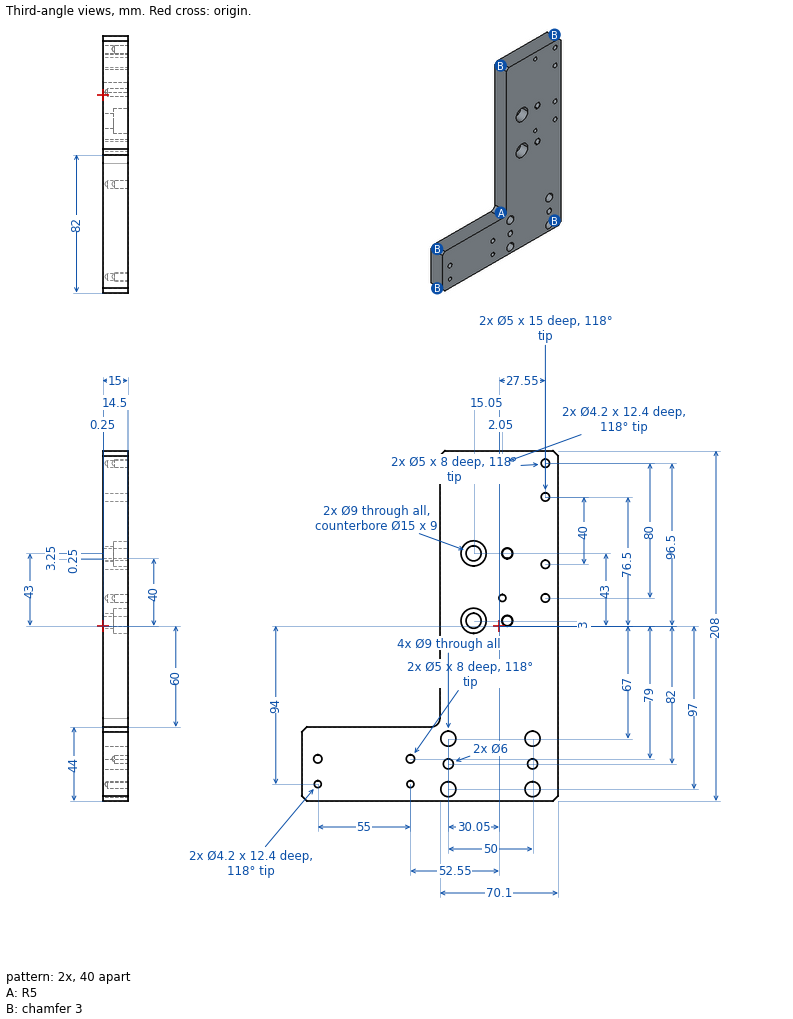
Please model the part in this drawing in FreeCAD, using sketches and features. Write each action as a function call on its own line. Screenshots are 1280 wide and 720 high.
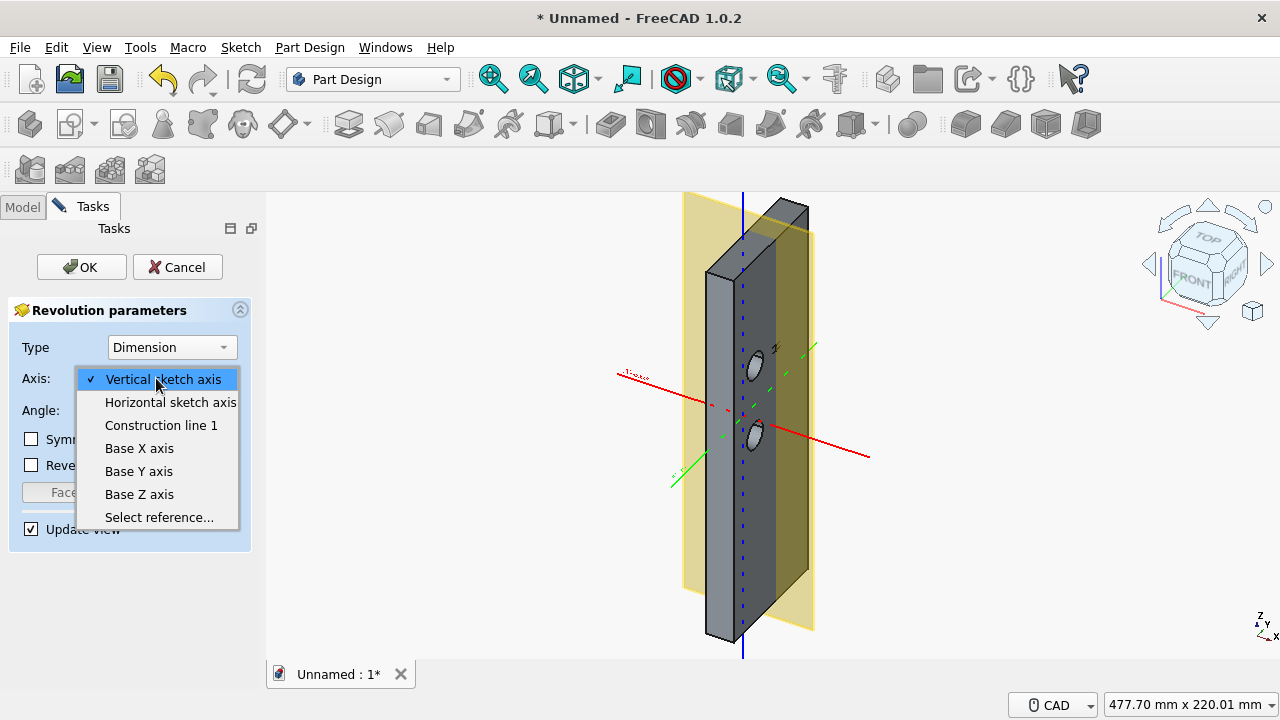
click(156, 426)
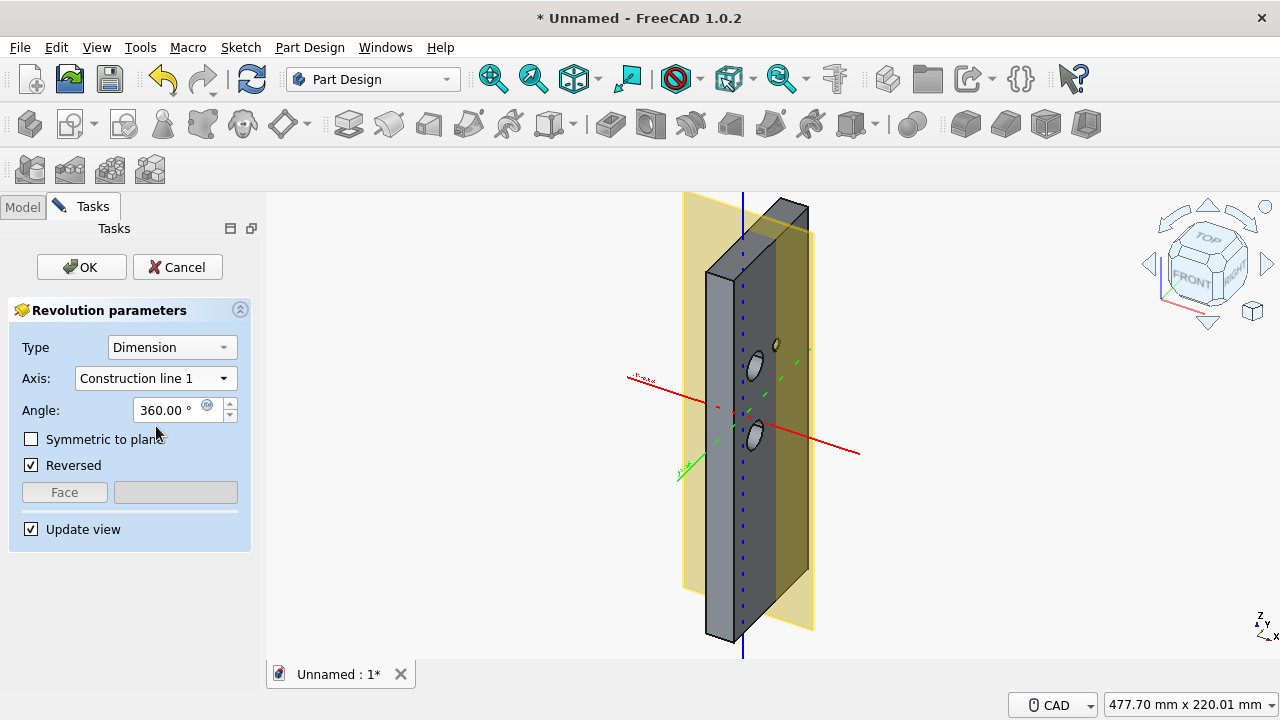
click(82, 267)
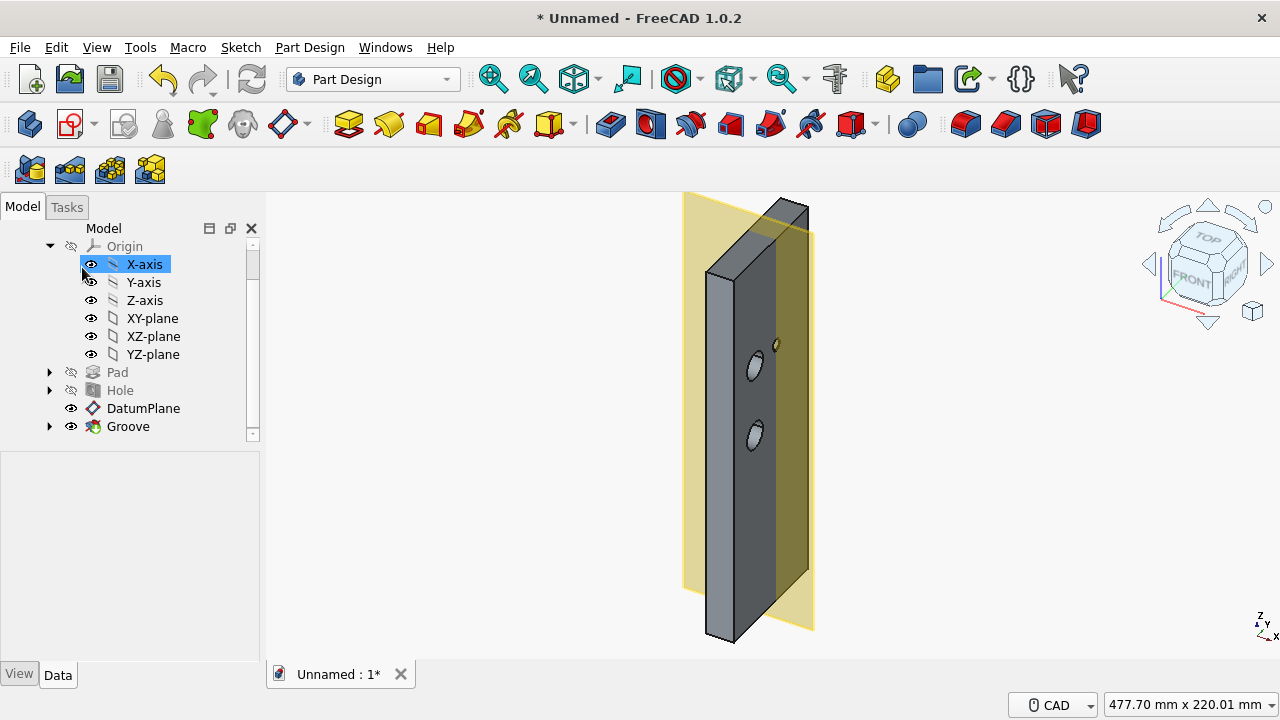
click(116, 408)
key(space)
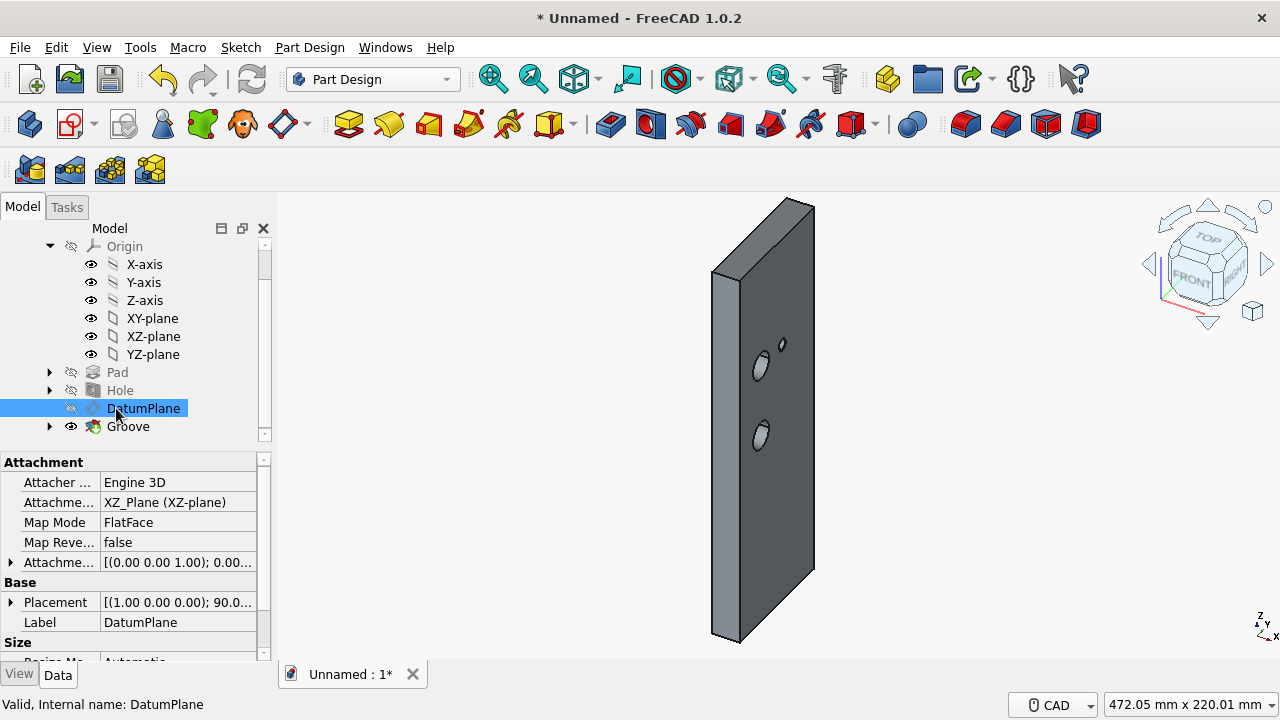
click(116, 426)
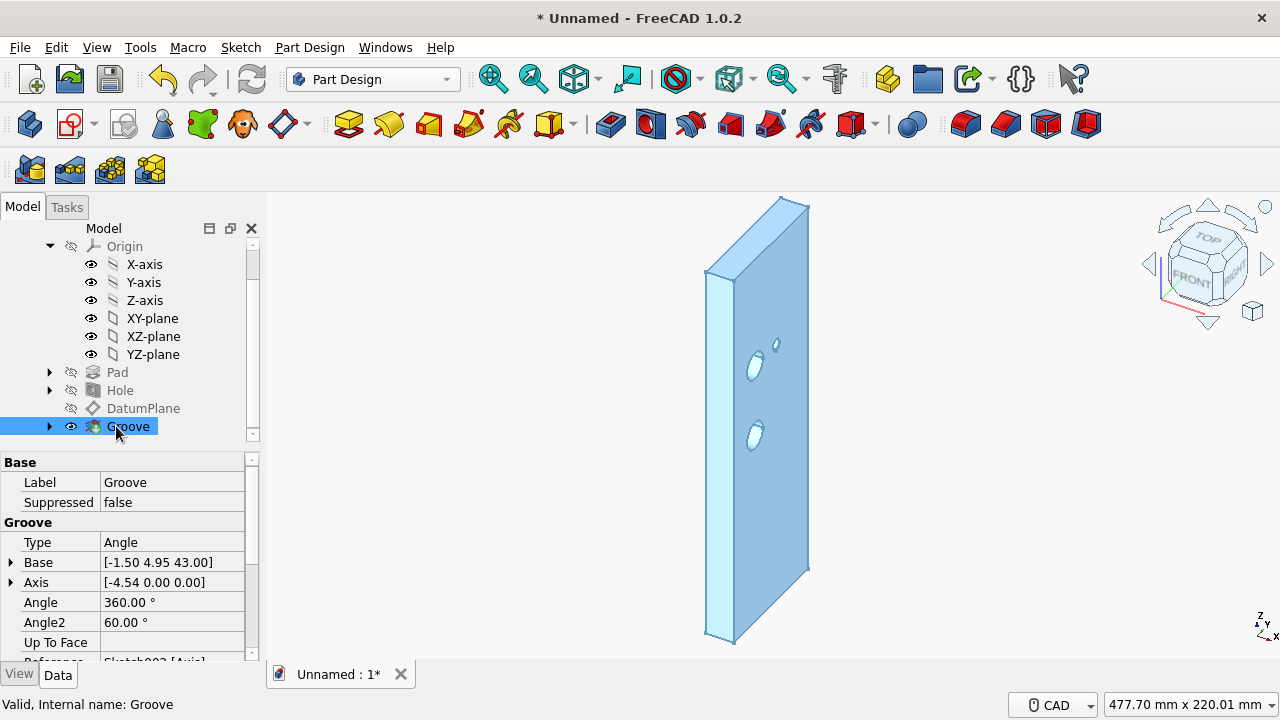
click(70, 170)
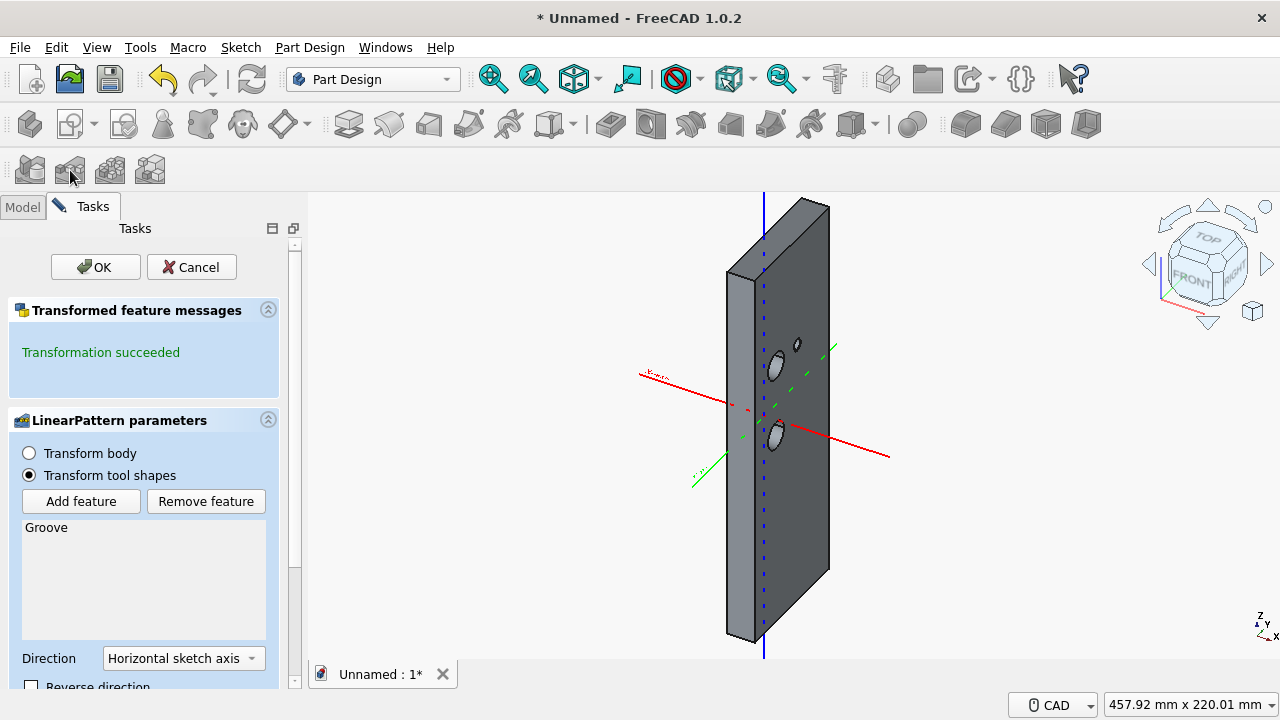
click(184, 658)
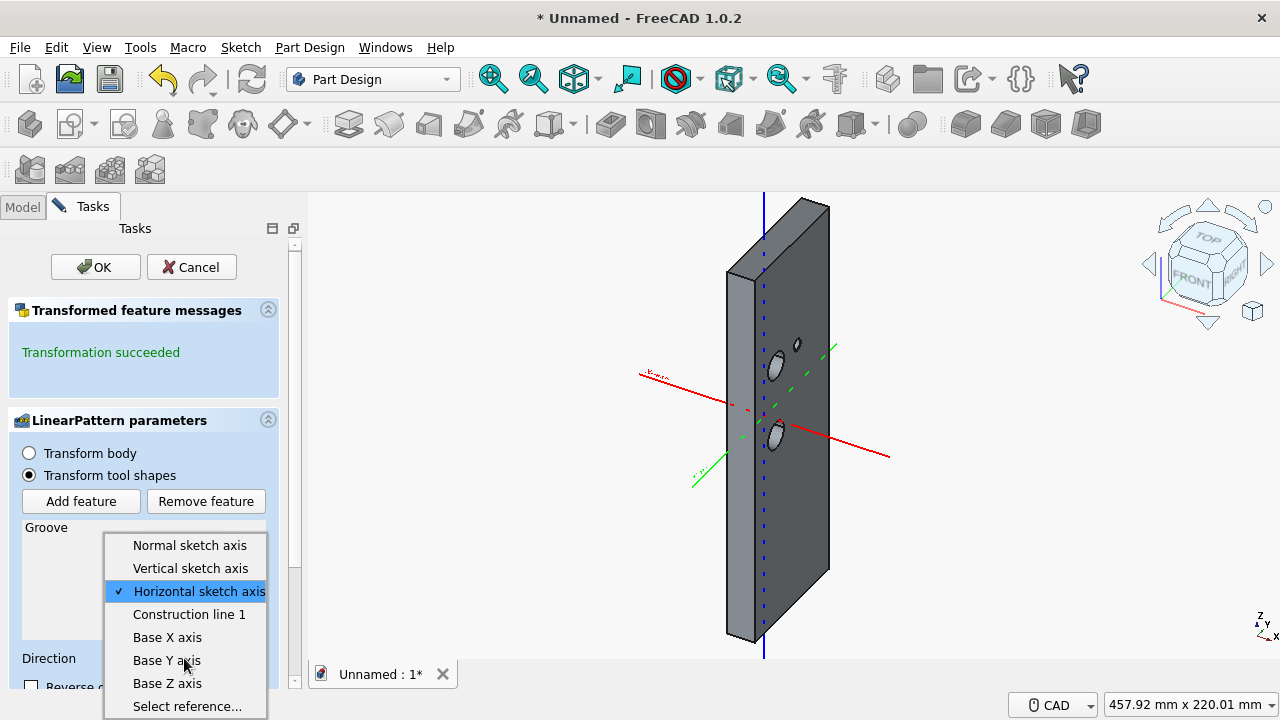
click(184, 684)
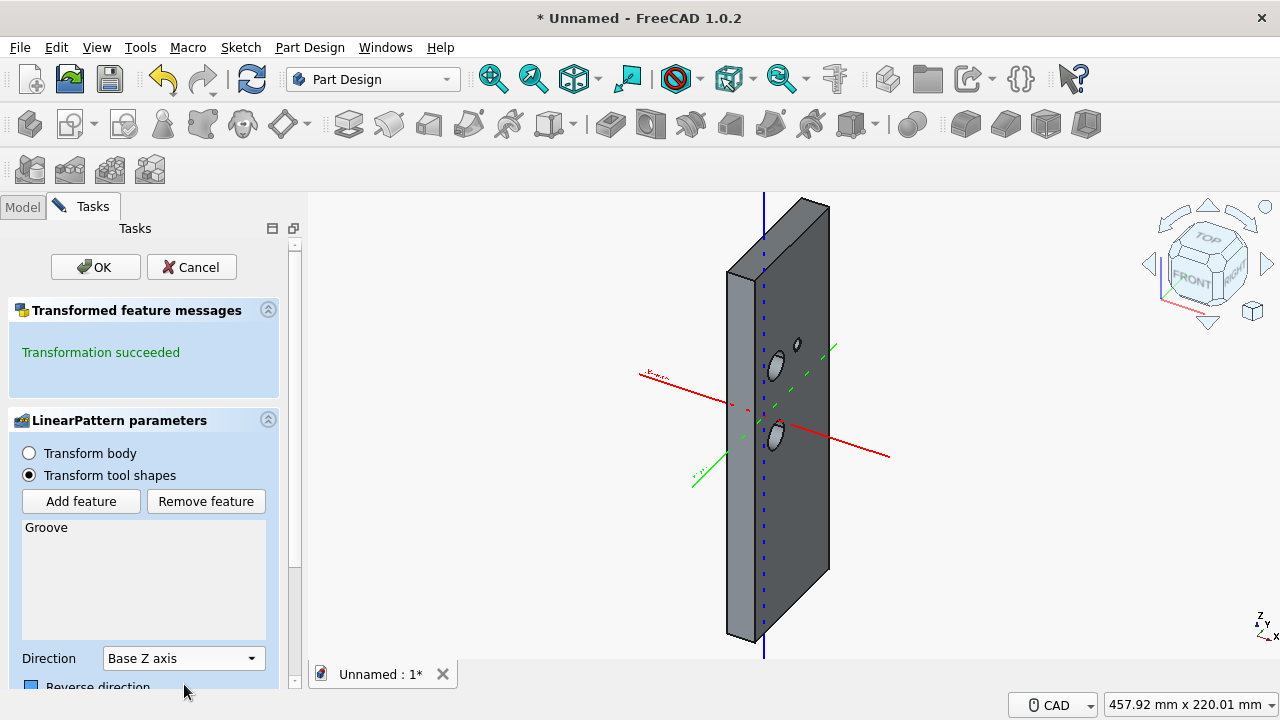
scroll(295, 463, down, 2)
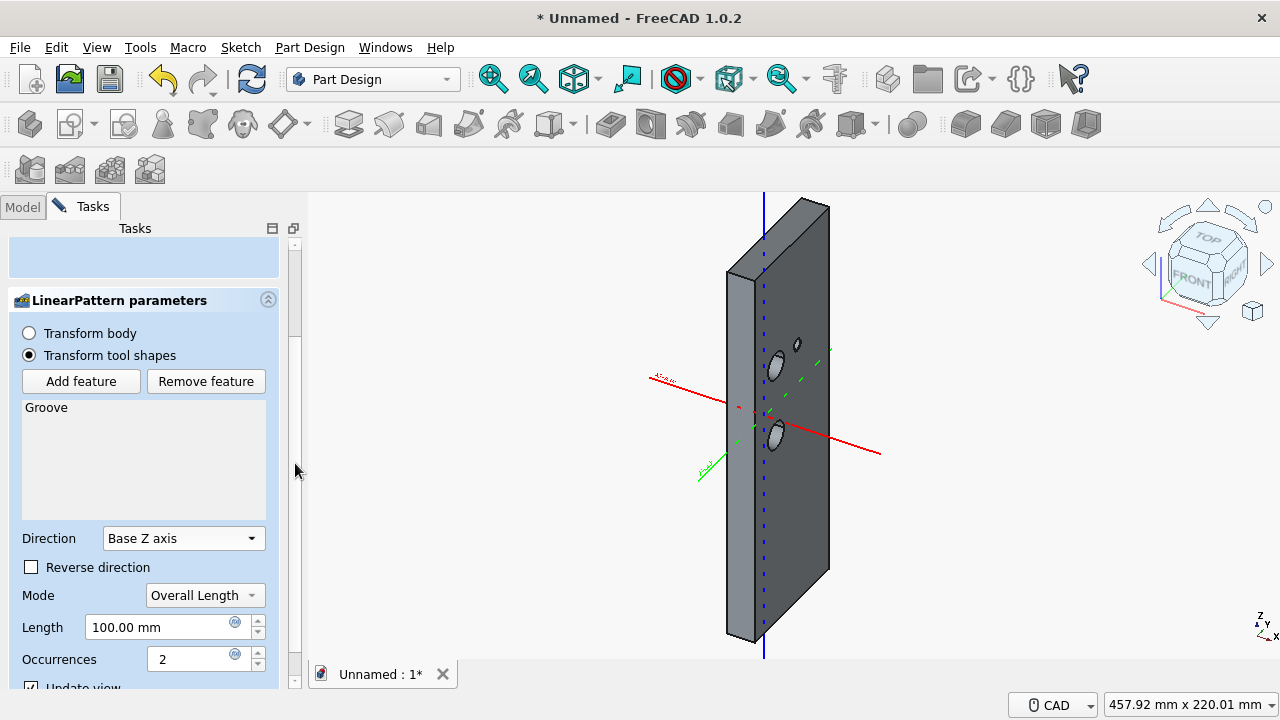
click(206, 596)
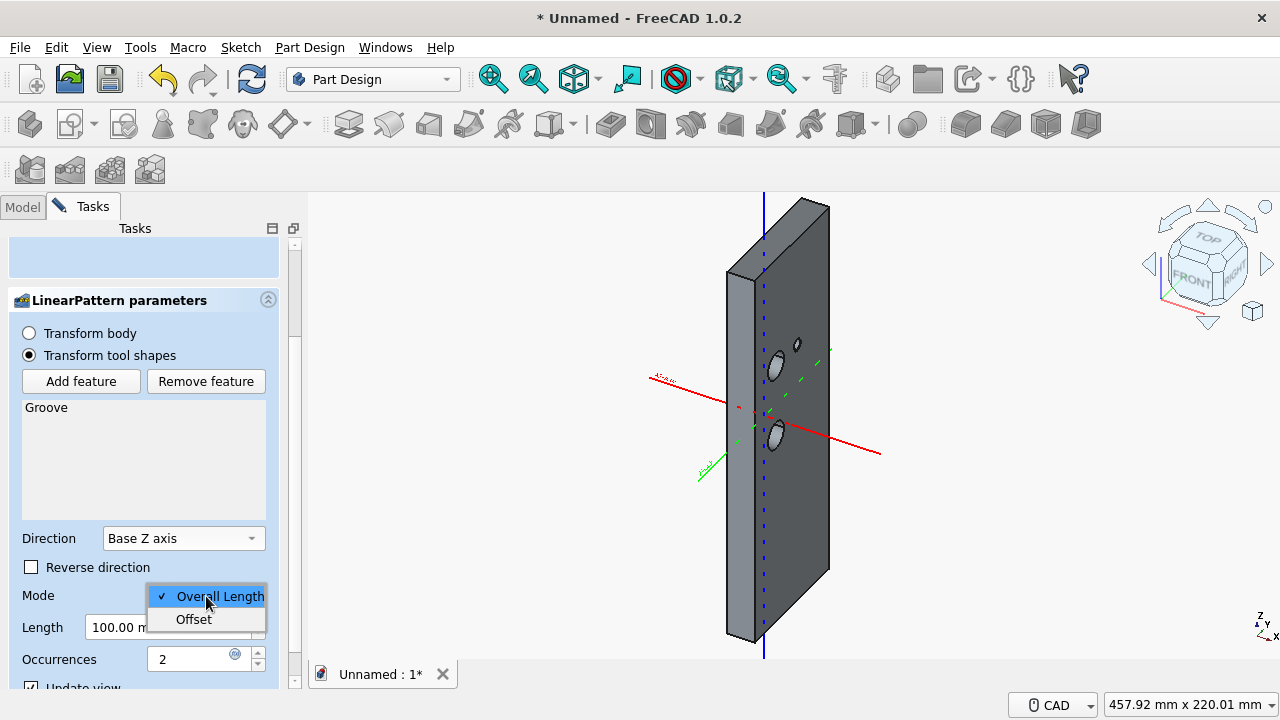
click(206, 620)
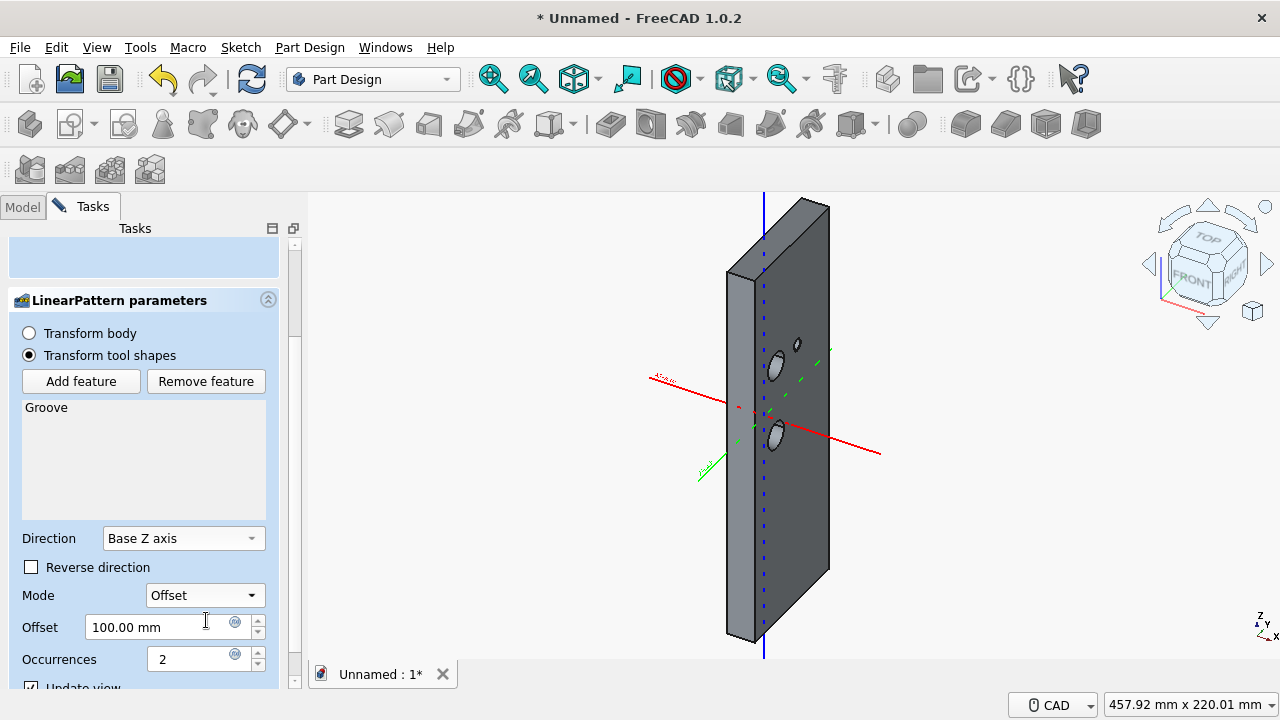
triple_click(168, 627)